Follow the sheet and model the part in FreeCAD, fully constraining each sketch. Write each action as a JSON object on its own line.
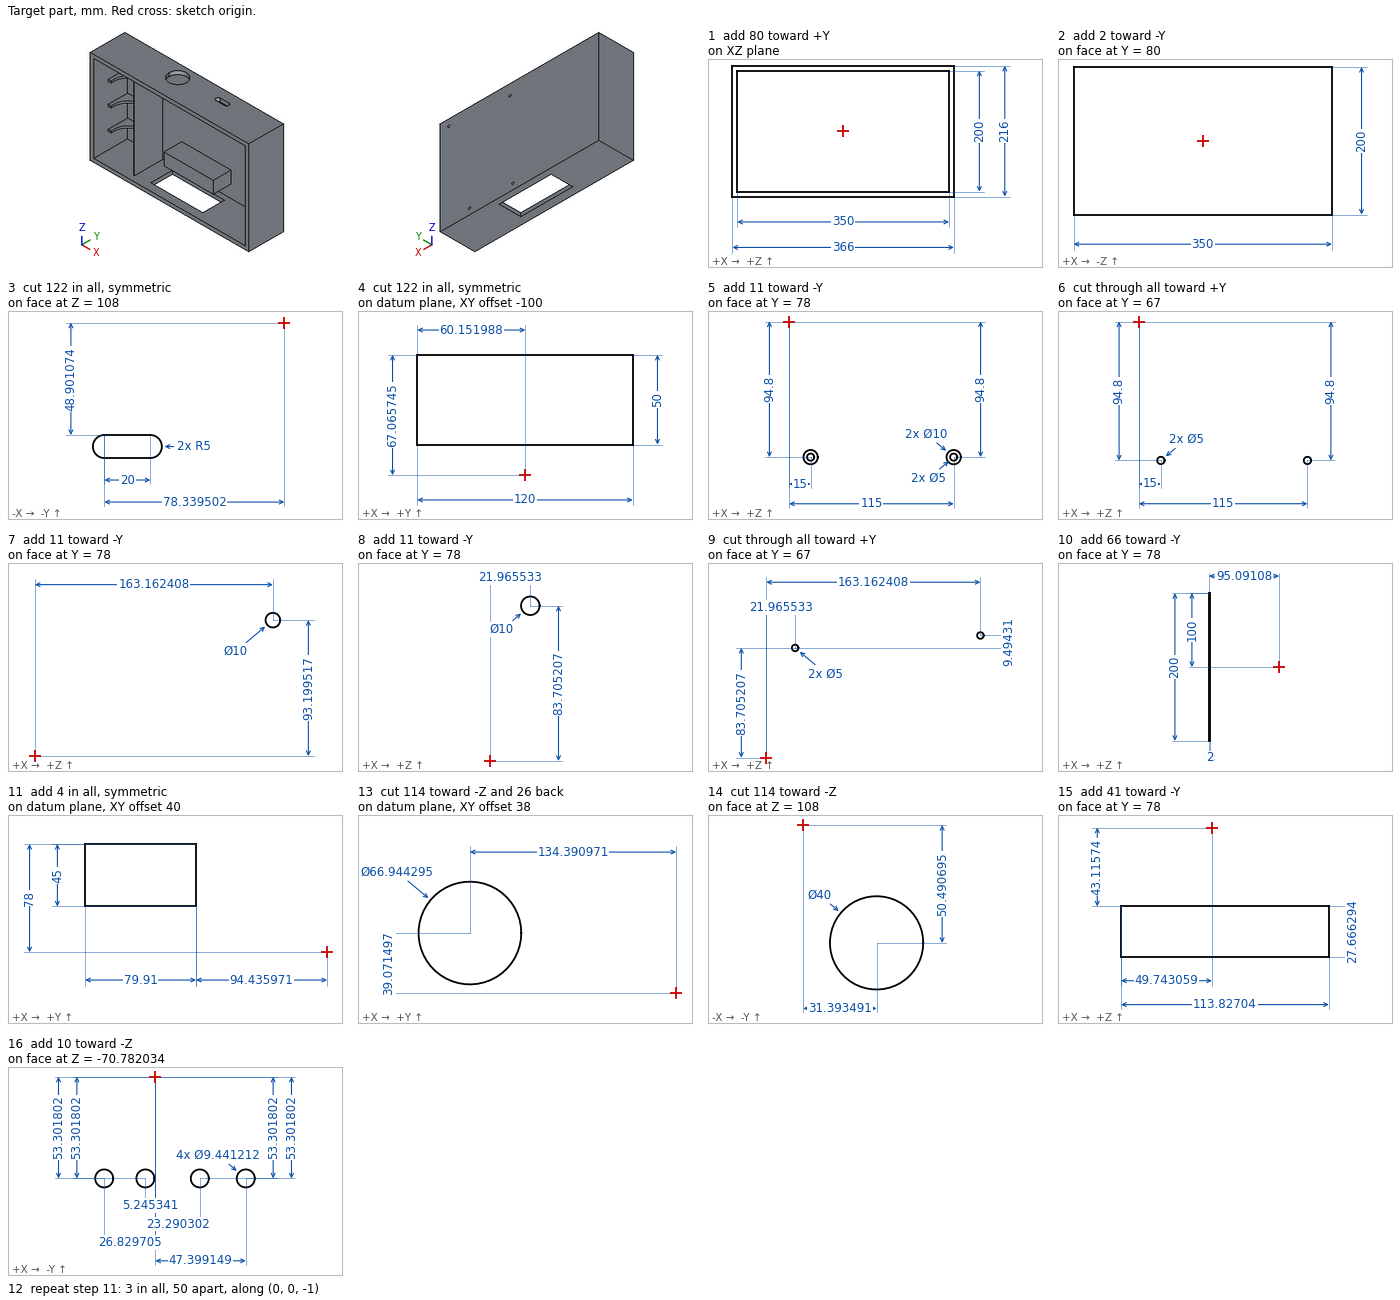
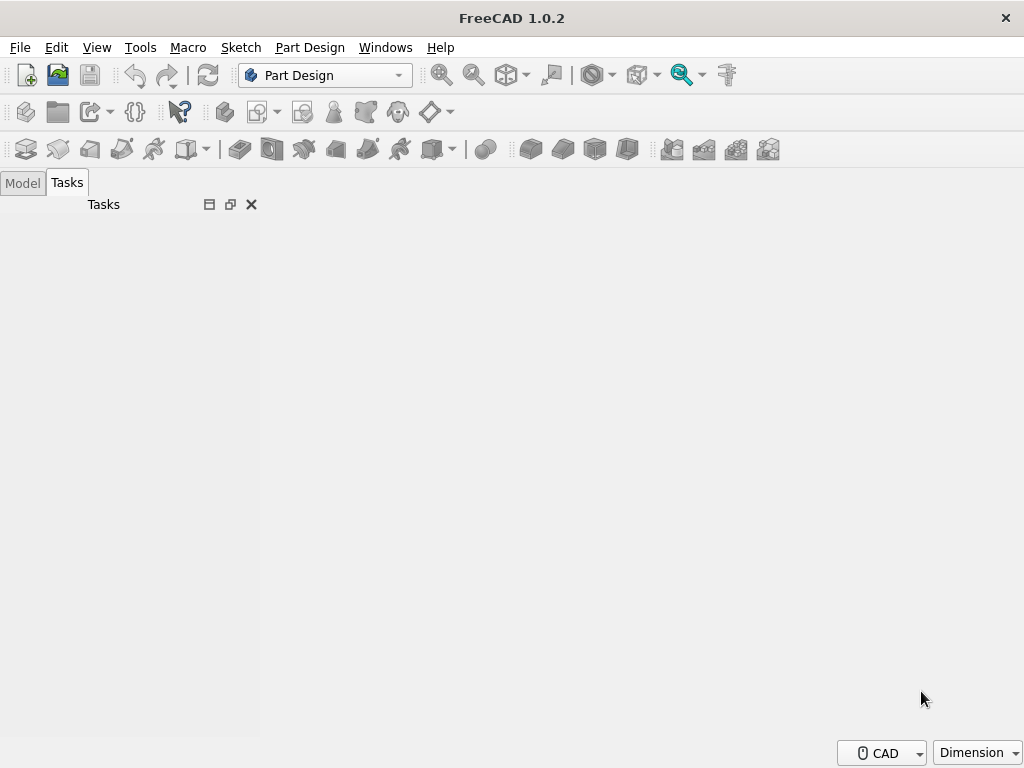
{"action": "left_click", "coordinate": [26, 76]}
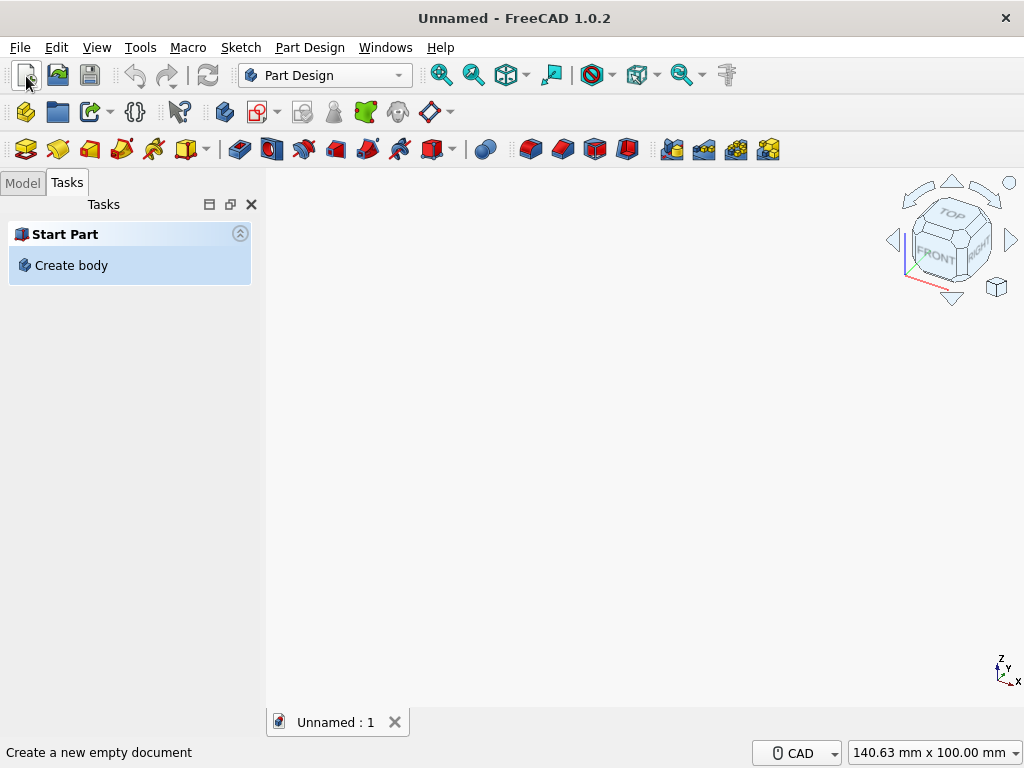
{"action": "left_click", "coordinate": [258, 112]}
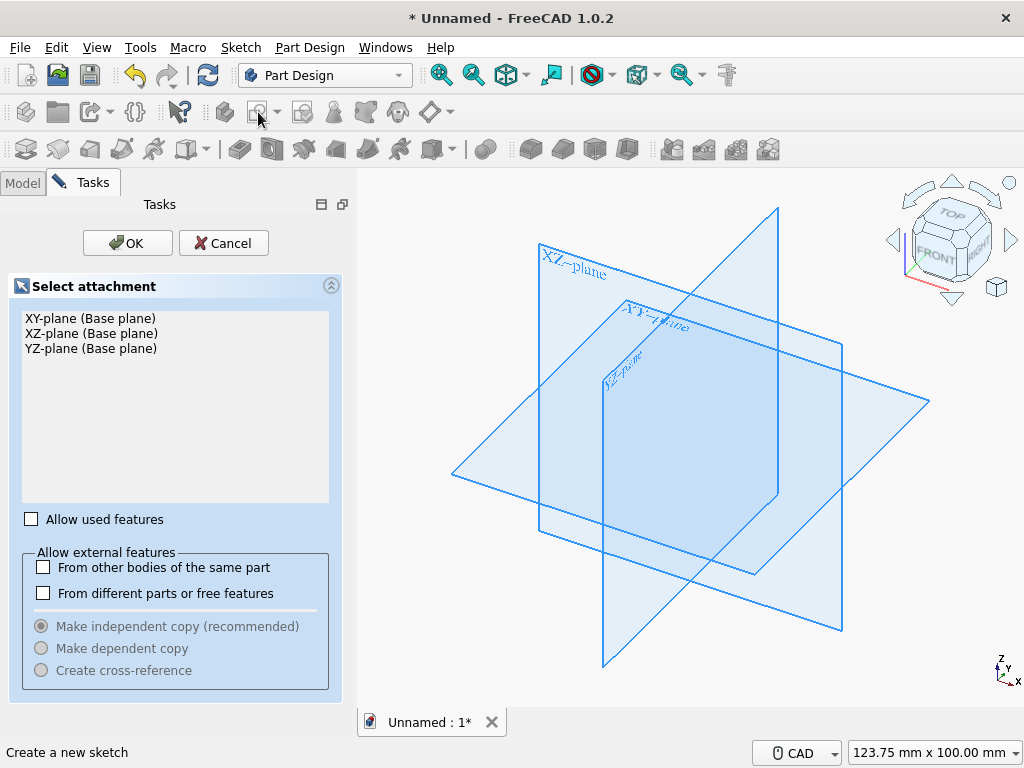
{"action": "left_click", "coordinate": [82, 334]}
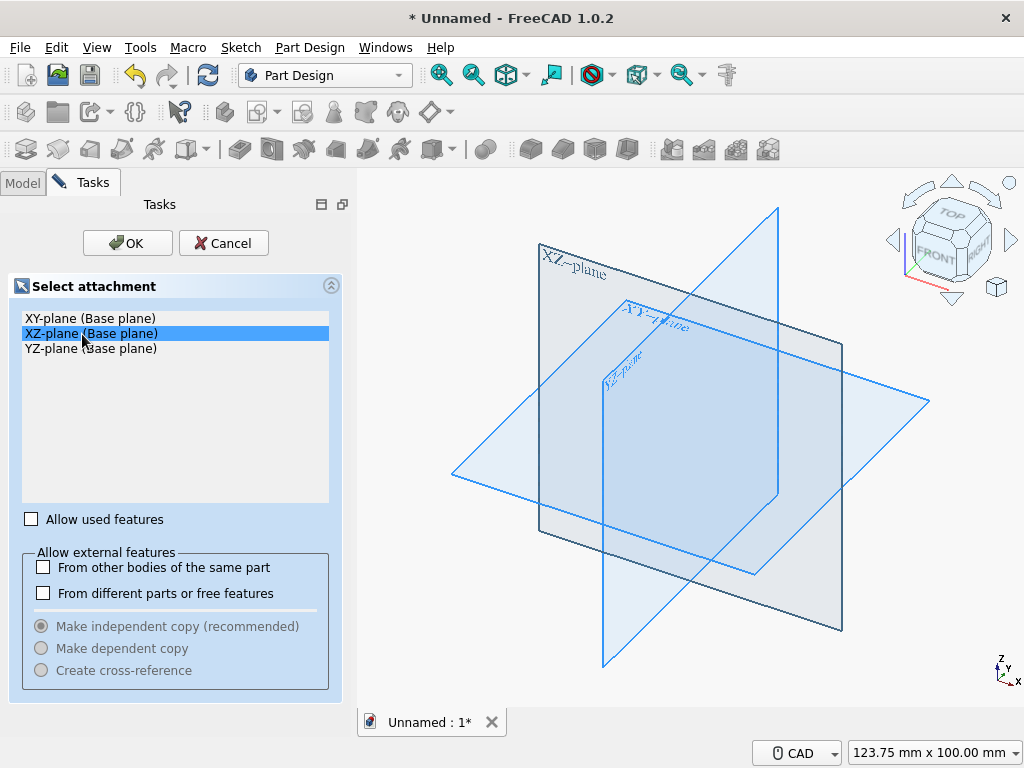
{"action": "left_click", "coordinate": [128, 243]}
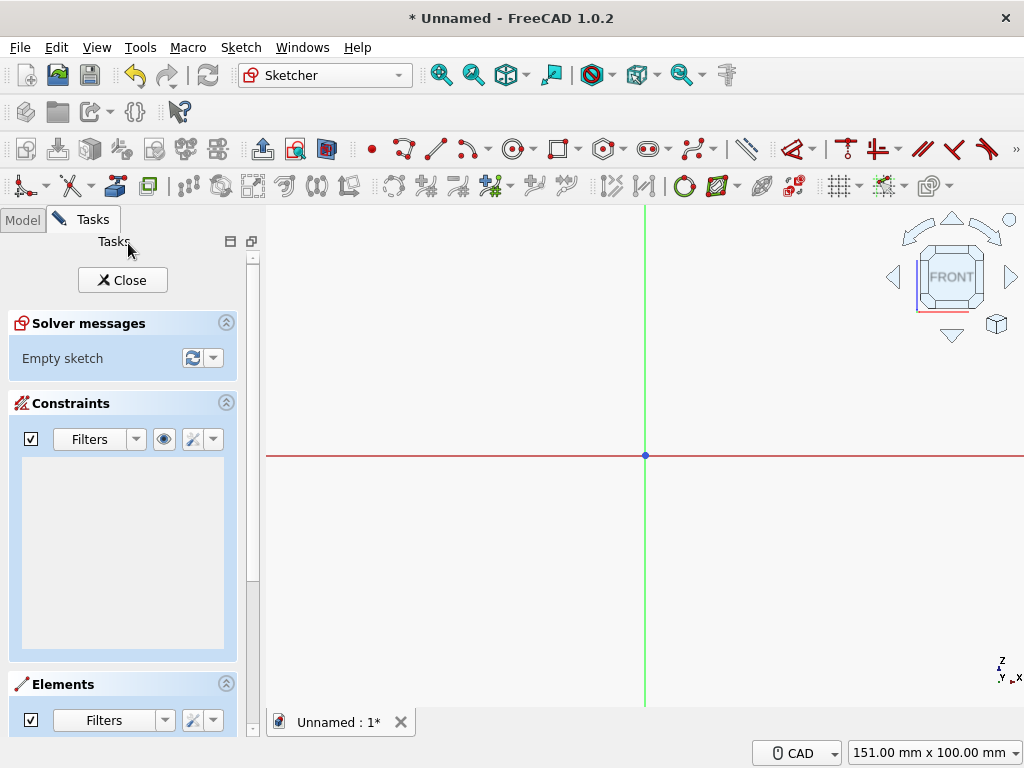
{"action": "scroll", "coordinate": [559, 456], "scroll_direction": "down", "scroll_amount": 8}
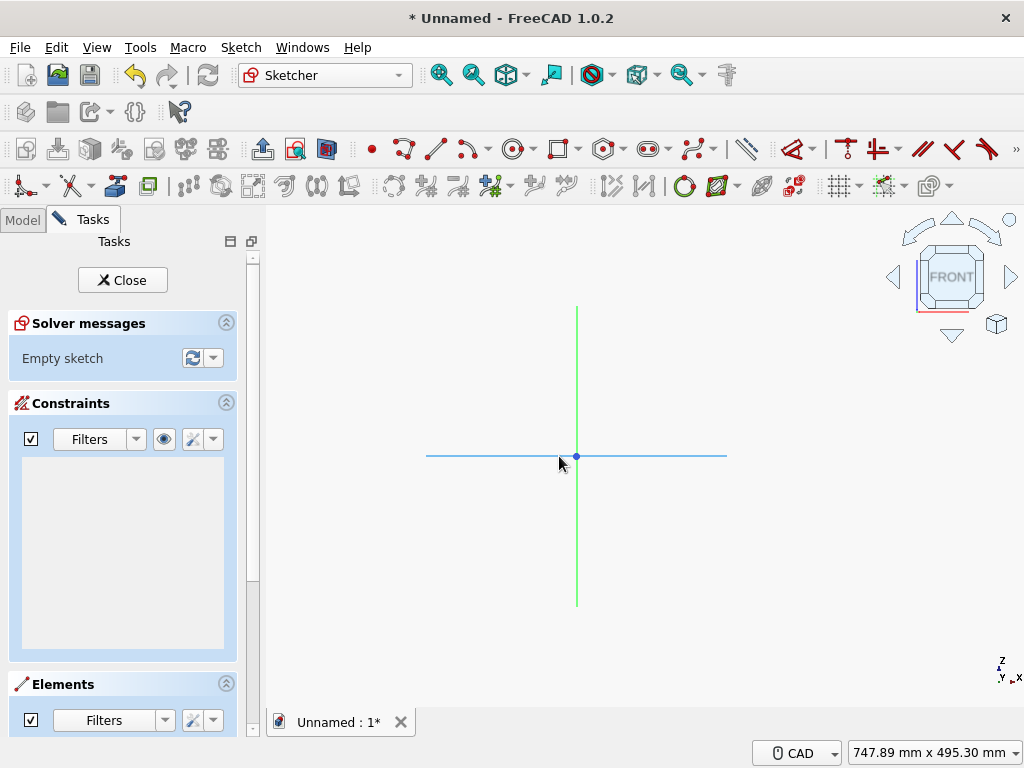
{"action": "key", "text": "g v"}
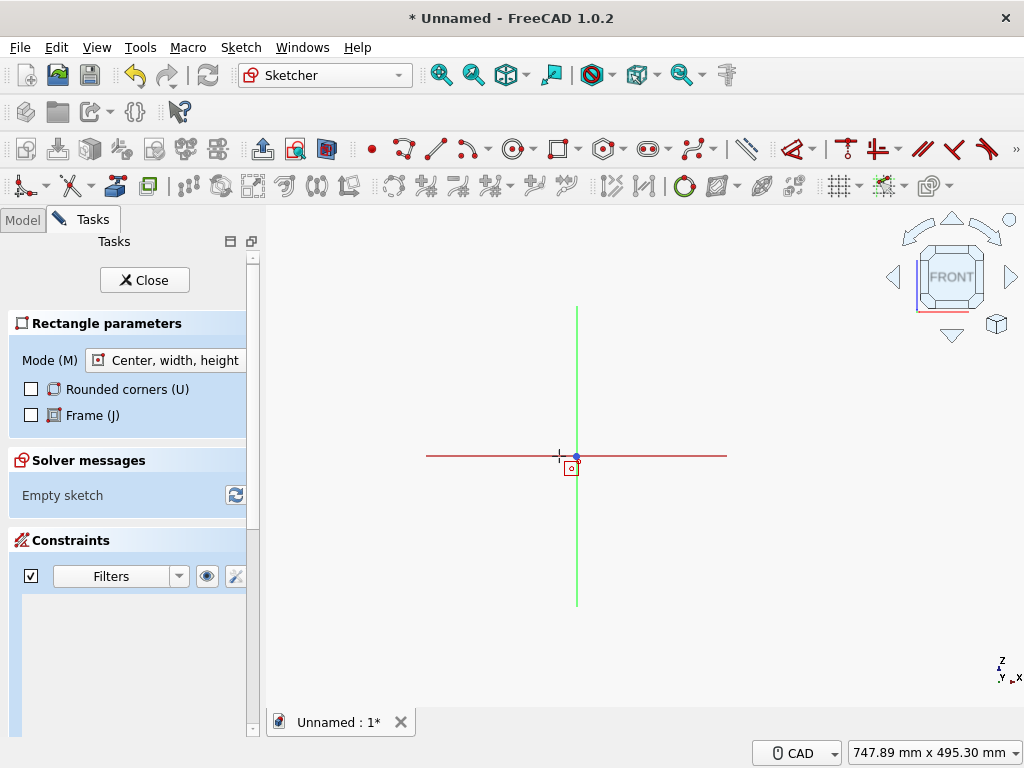
{"action": "left_click", "coordinate": [577, 456]}
{"action": "mouse_move", "coordinate": [762, 347]}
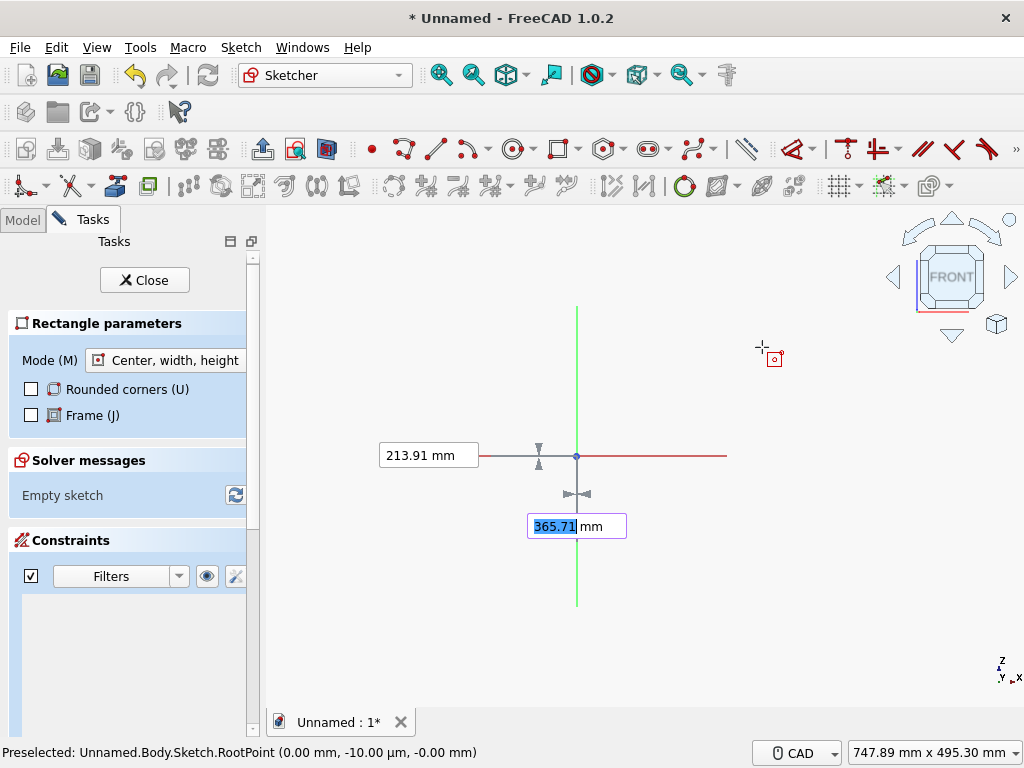
{"action": "type", "text": "366"}
{"action": "key", "text": "Tab"}
{"action": "type", "text": "216"}
{"action": "key", "text": "Return"}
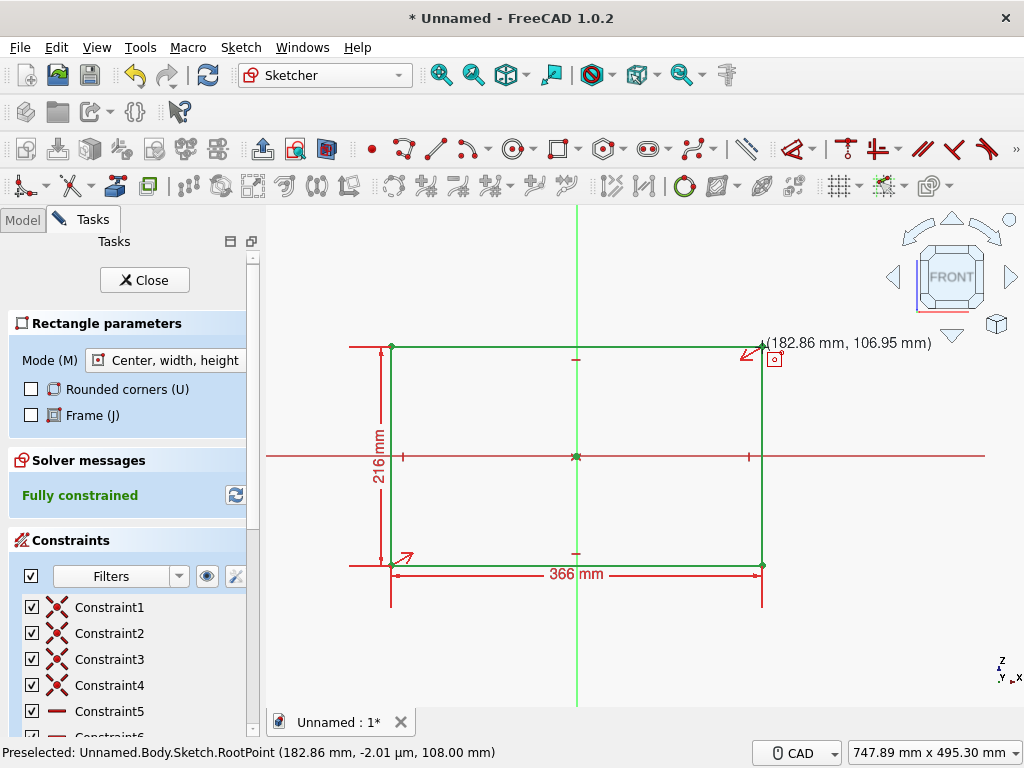
{"action": "left_click", "coordinate": [577, 456]}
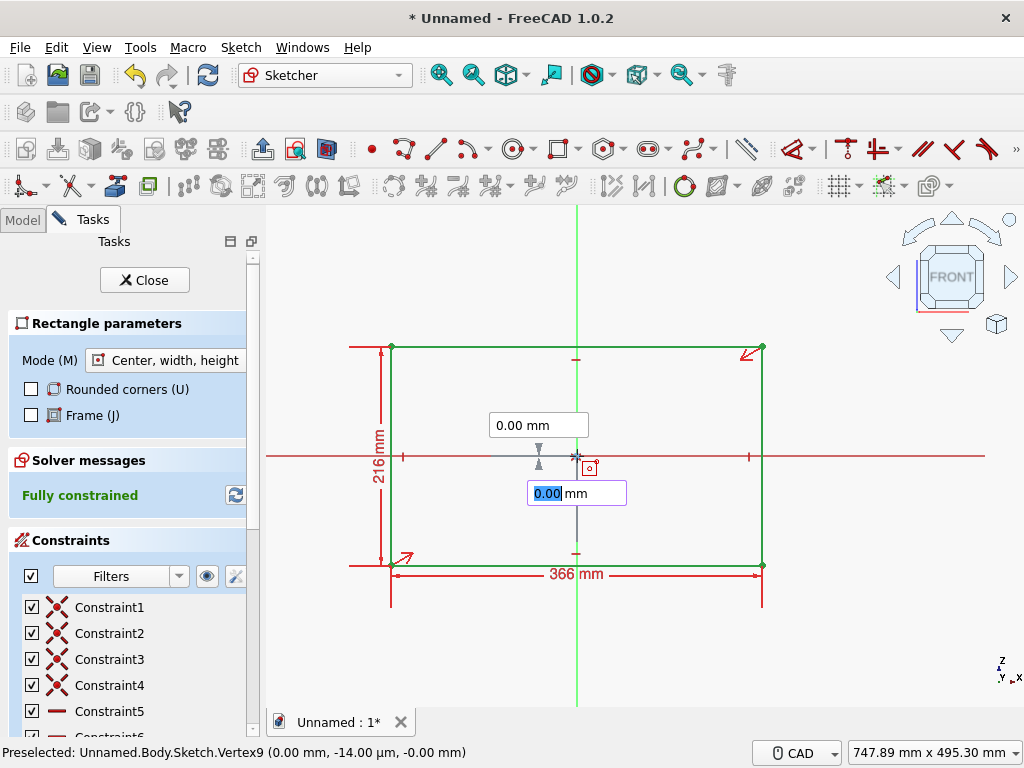
{"action": "scroll", "coordinate": [754, 355], "scroll_direction": "up", "scroll_amount": 4}
{"action": "mouse_move", "coordinate": [753, 355]}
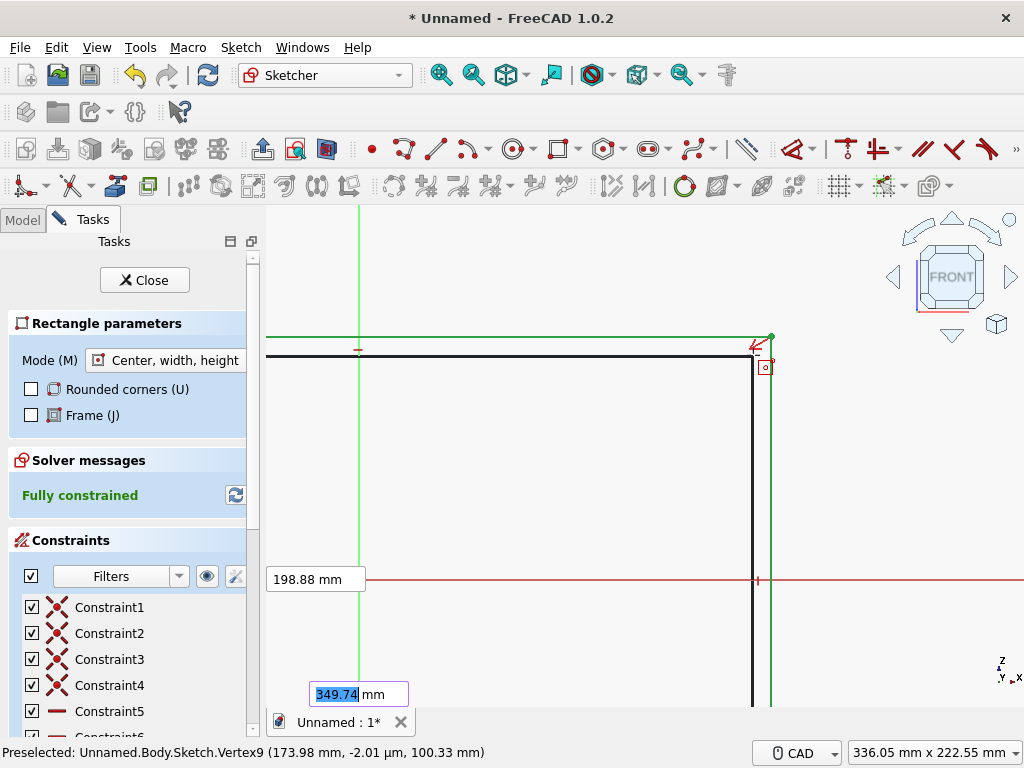
{"action": "type", "text": "350"}
{"action": "key", "text": "Tab"}
{"action": "type", "text": "200"}
{"action": "key", "text": "Return"}
{"action": "key", "text": "Escape"}